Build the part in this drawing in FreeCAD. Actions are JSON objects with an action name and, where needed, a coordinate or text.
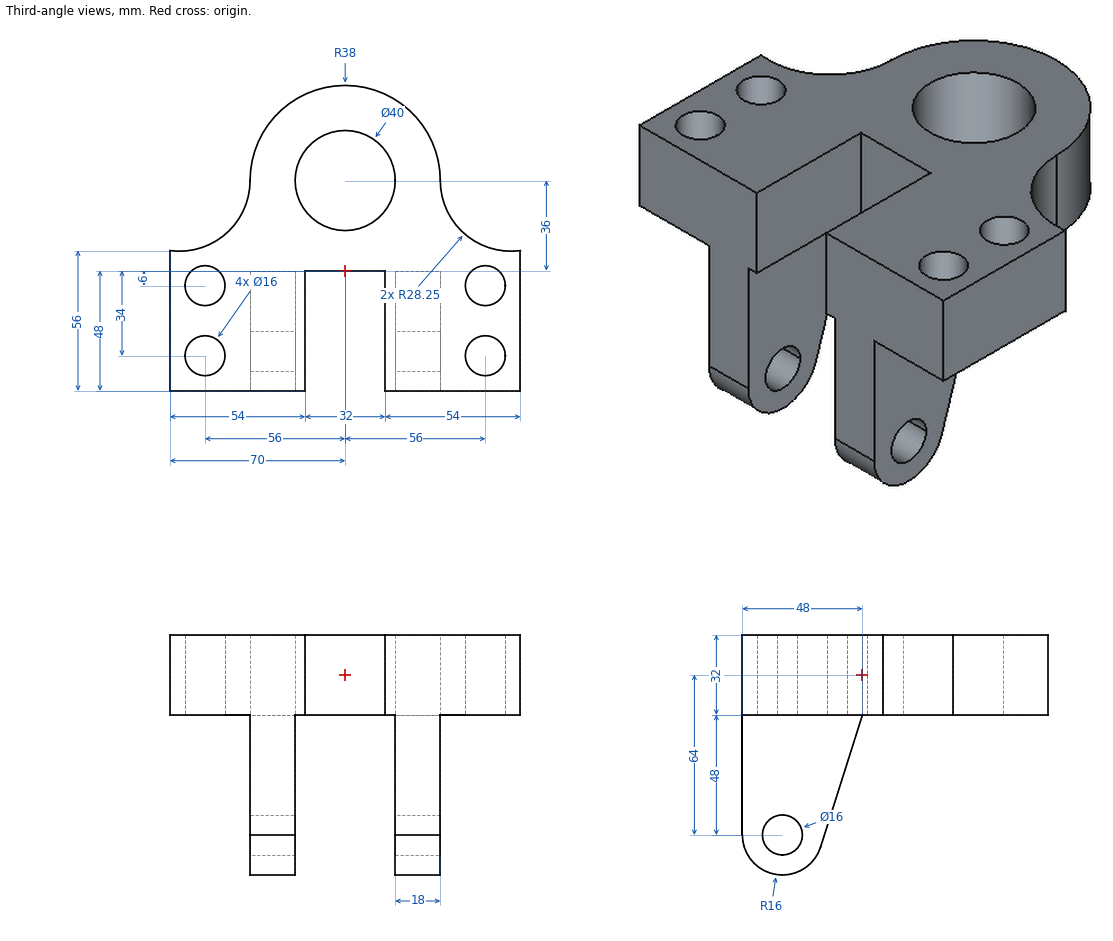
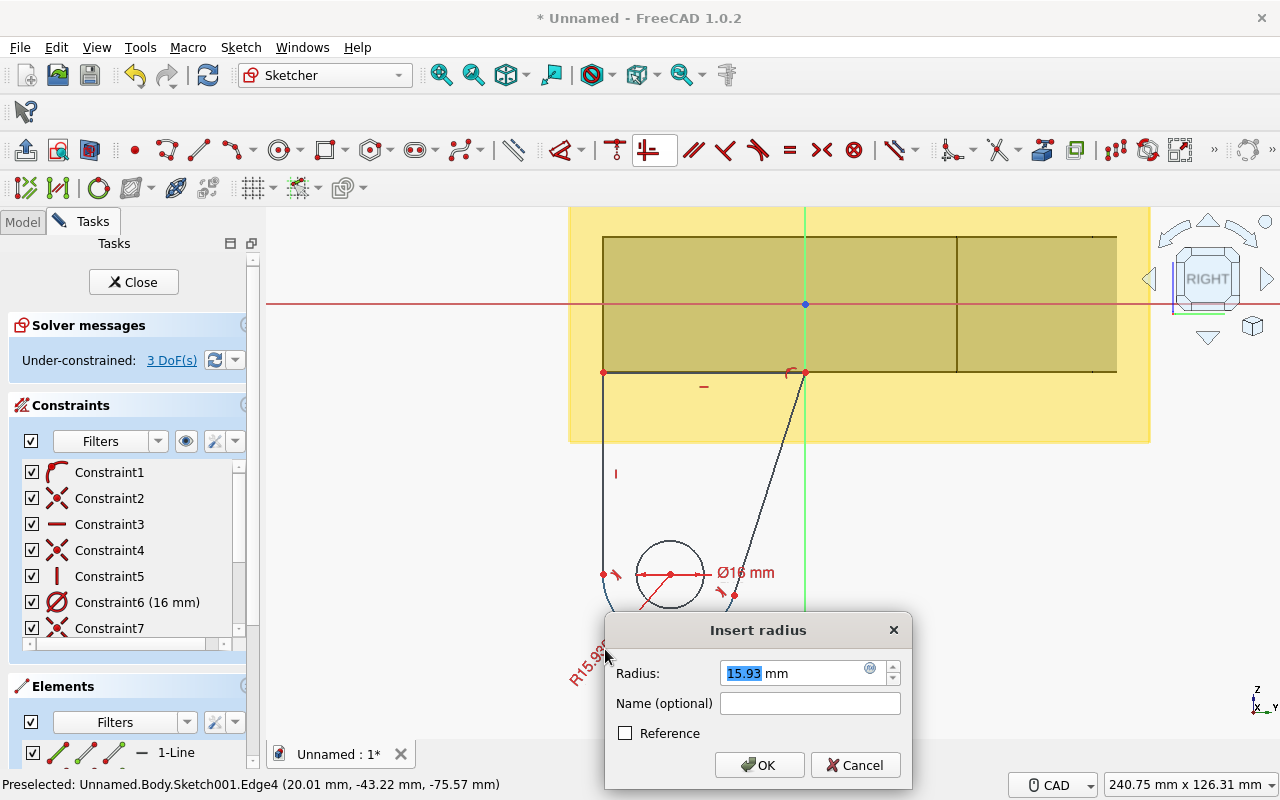
{"action": "type", "text": "16"}
{"action": "key", "text": "Return"}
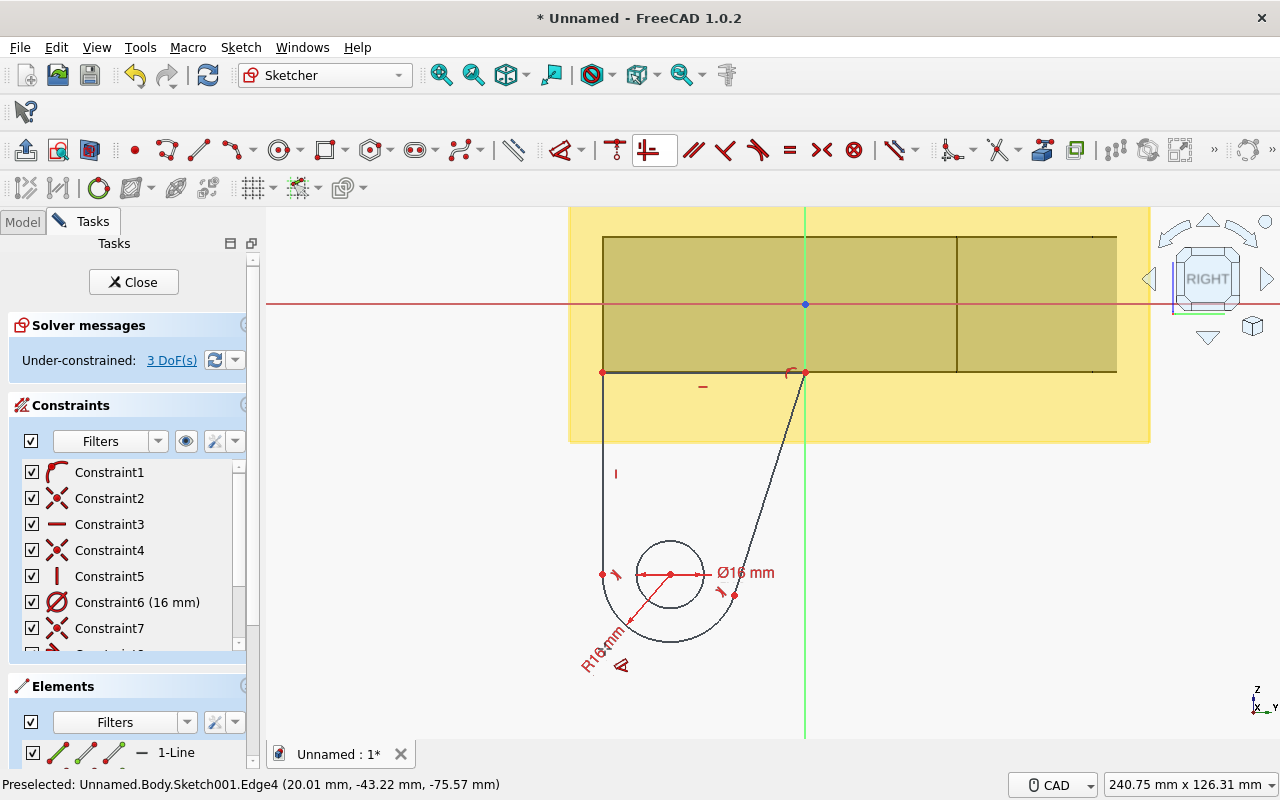
{"action": "left_click", "coordinate": [744, 373]}
{"action": "left_click", "coordinate": [704, 339]}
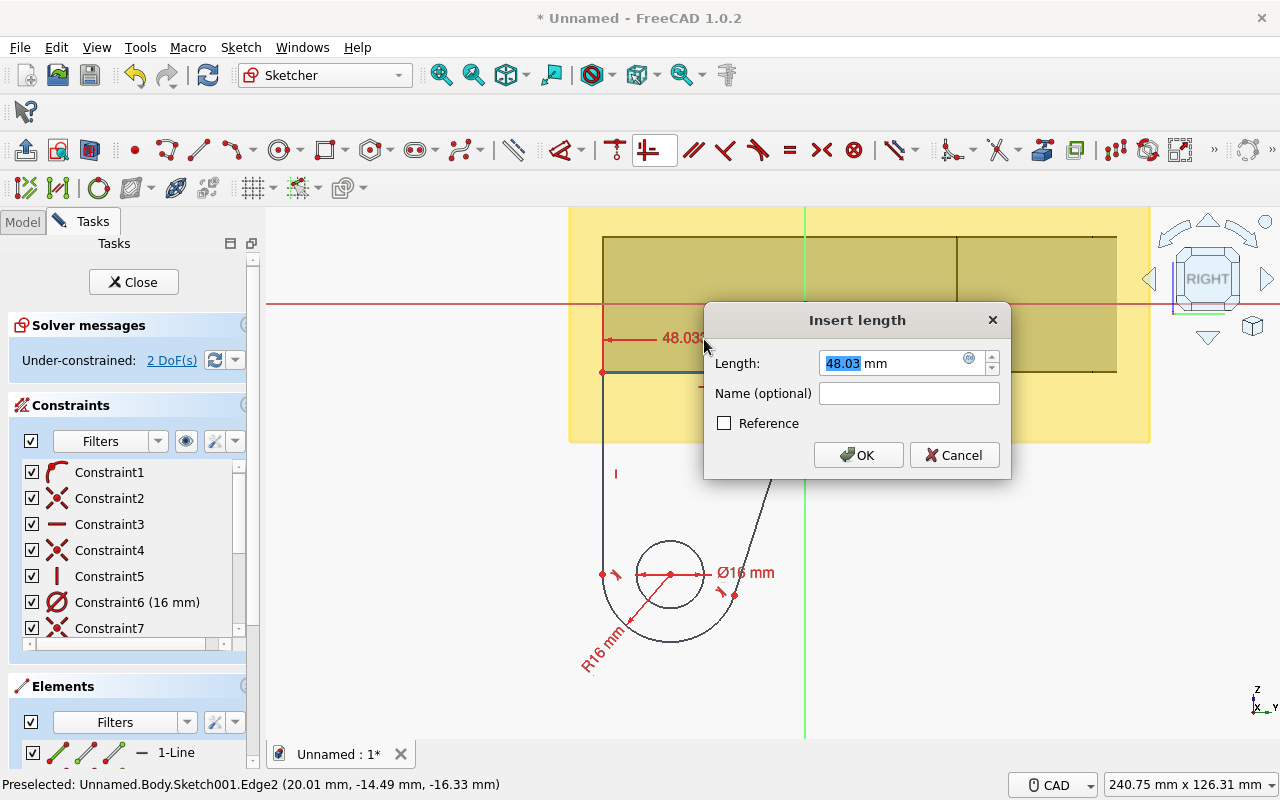
{"action": "type", "text": "48"}
{"action": "key", "text": "Return"}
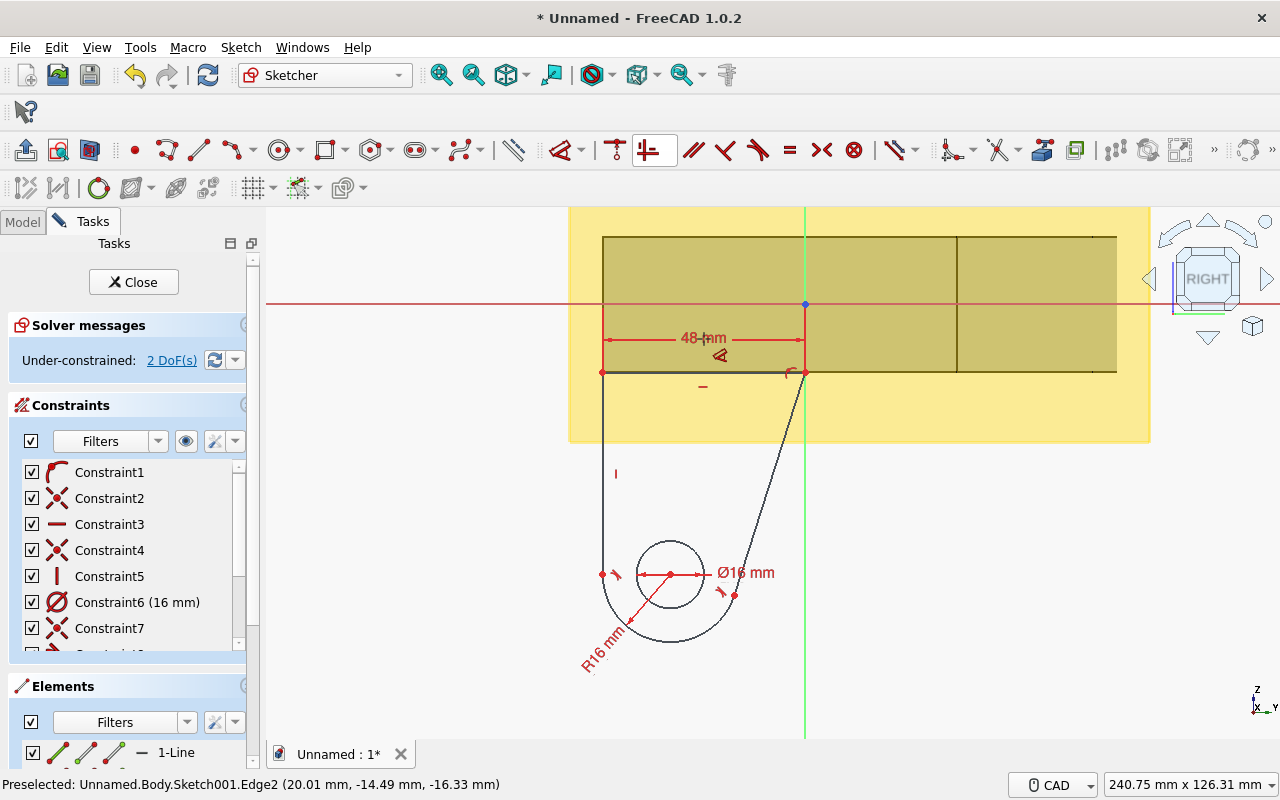
{"action": "left_click", "coordinate": [603, 434]}
{"action": "left_click", "coordinate": [569, 474]}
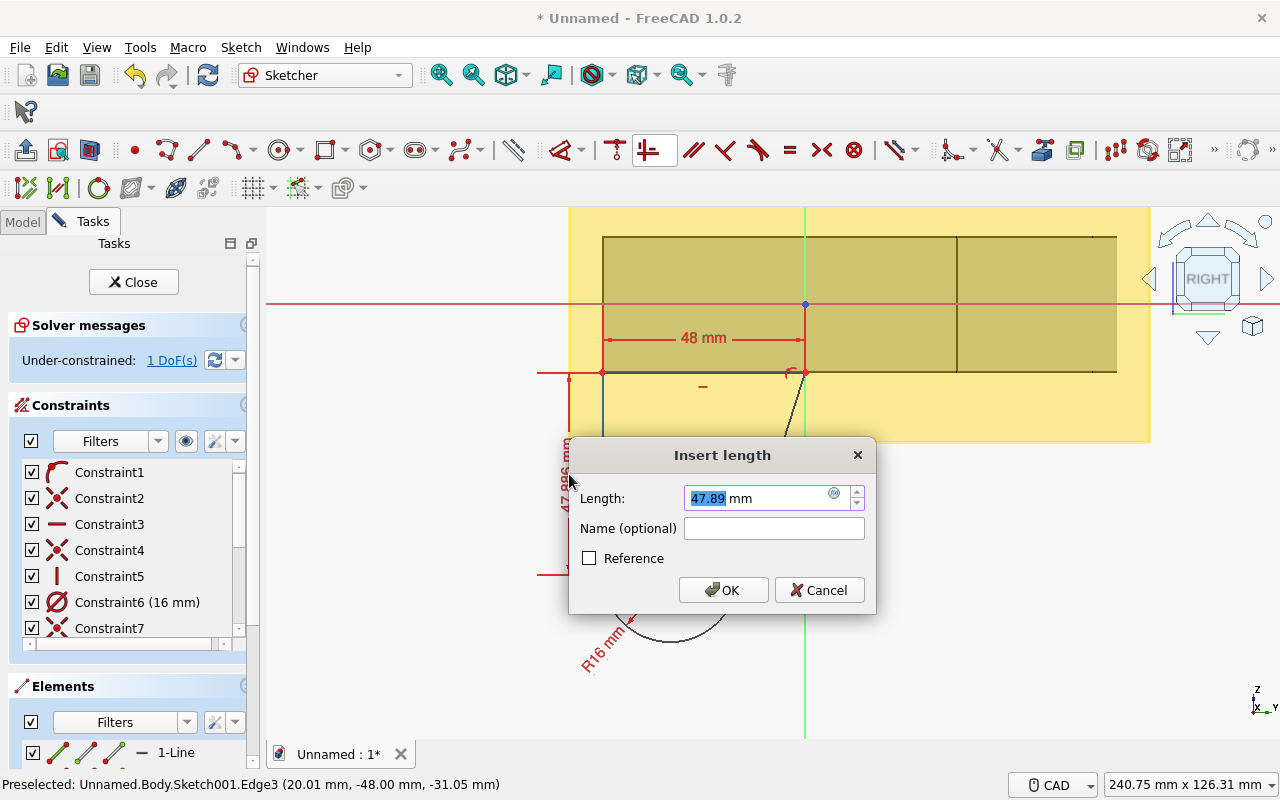
{"action": "type", "text": "48"}
{"action": "key", "text": "Return"}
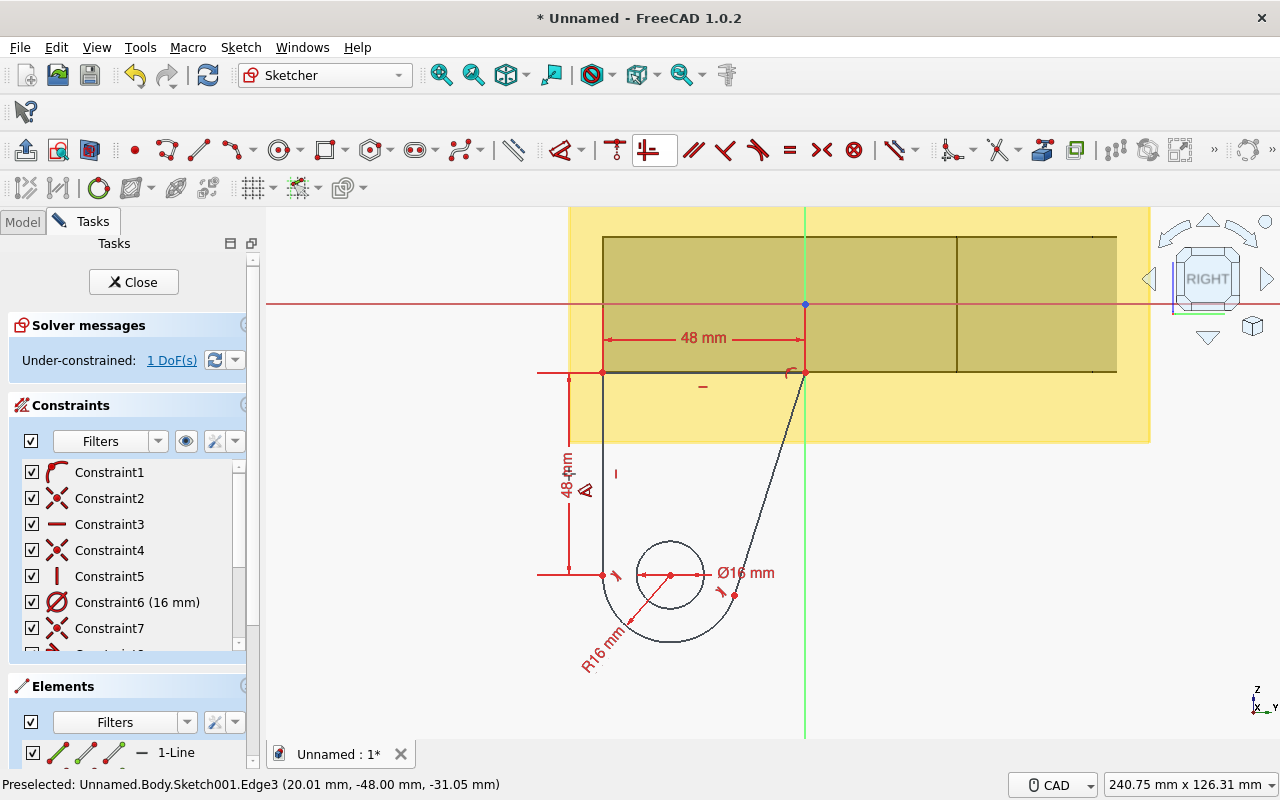
{"action": "left_click", "coordinate": [670, 575]}
{"action": "left_click", "coordinate": [839, 440]}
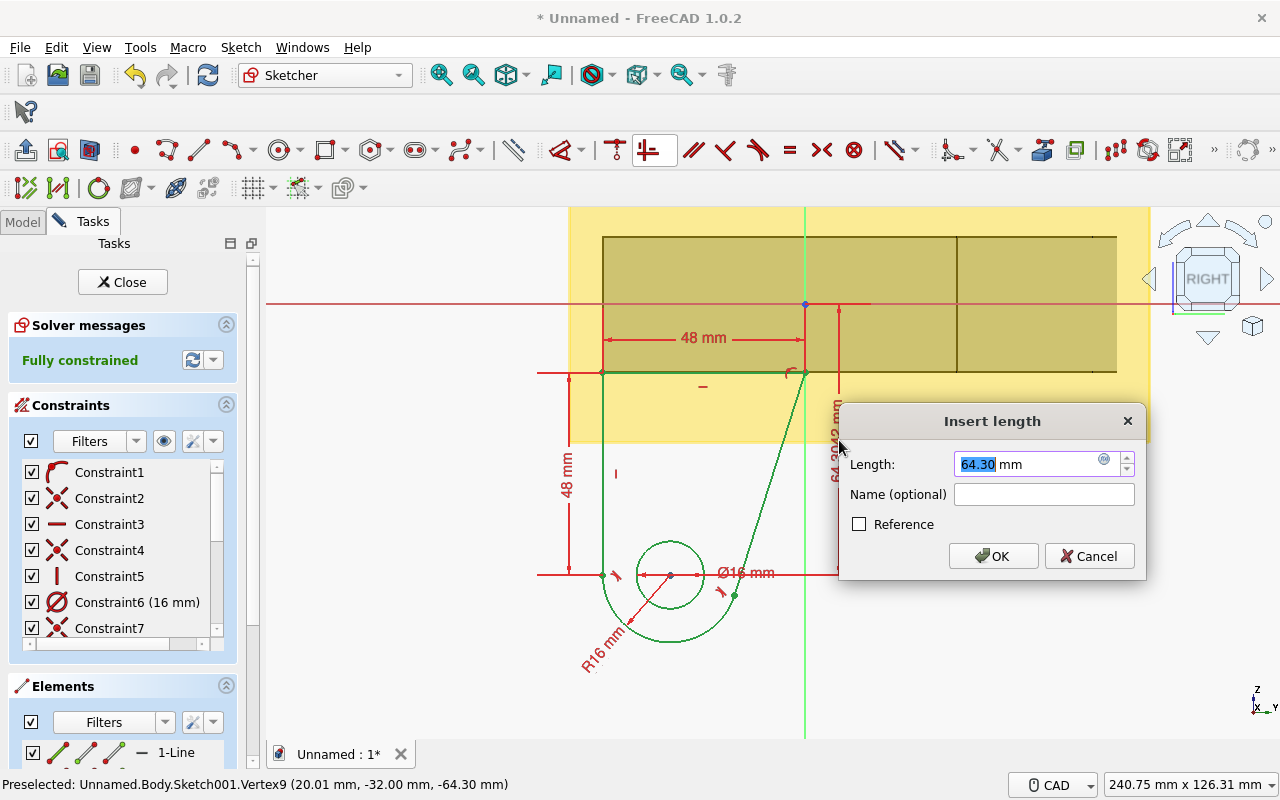
{"action": "type", "text": "64"}
{"action": "key", "text": "Return"}
{"action": "key", "text": "Escape"}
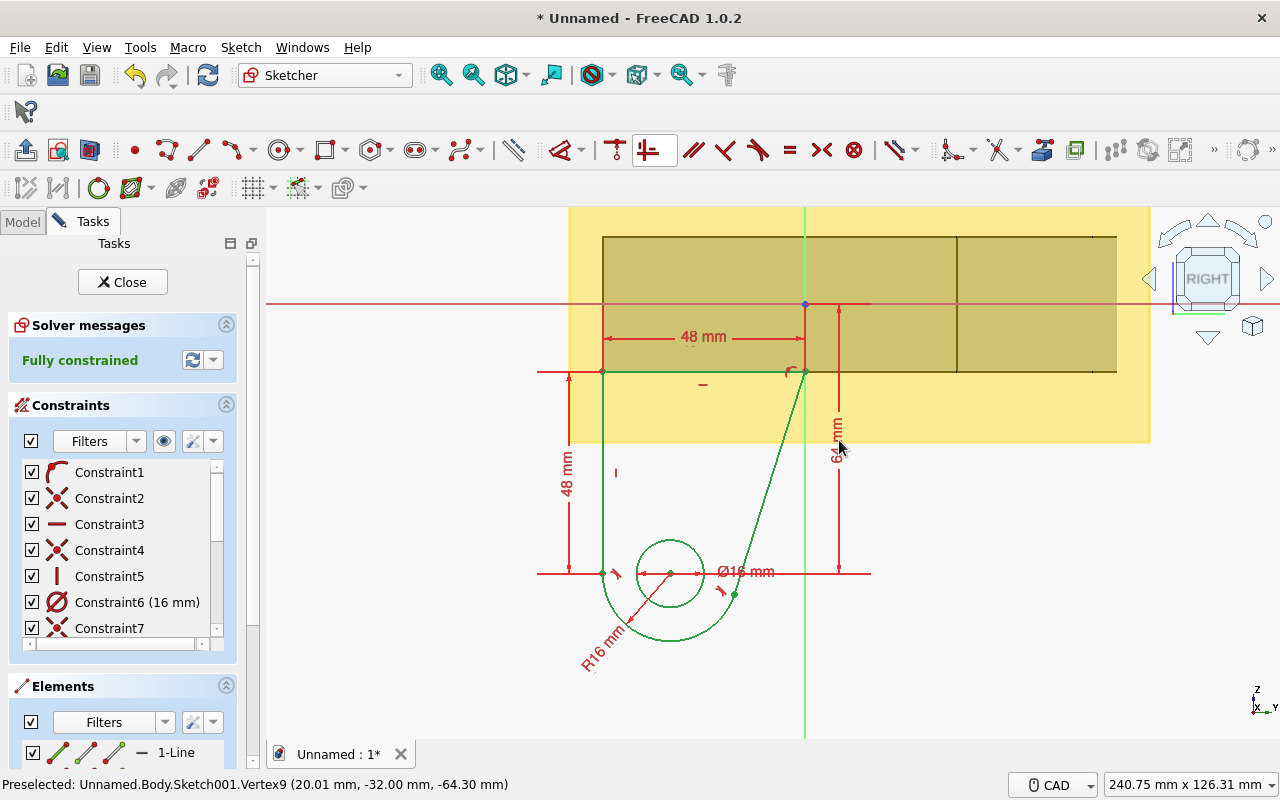
{"action": "left_click", "coordinate": [123, 282]}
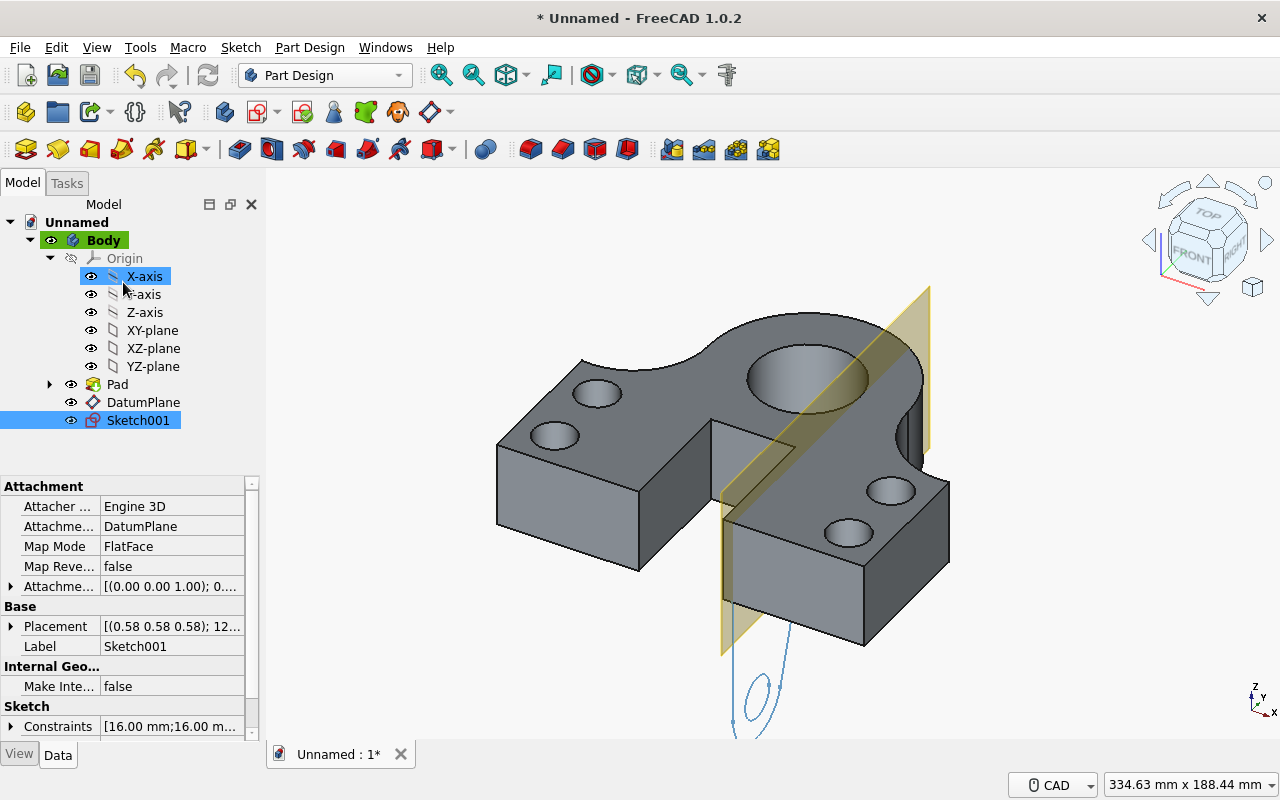
{"action": "left_click", "coordinate": [26, 150]}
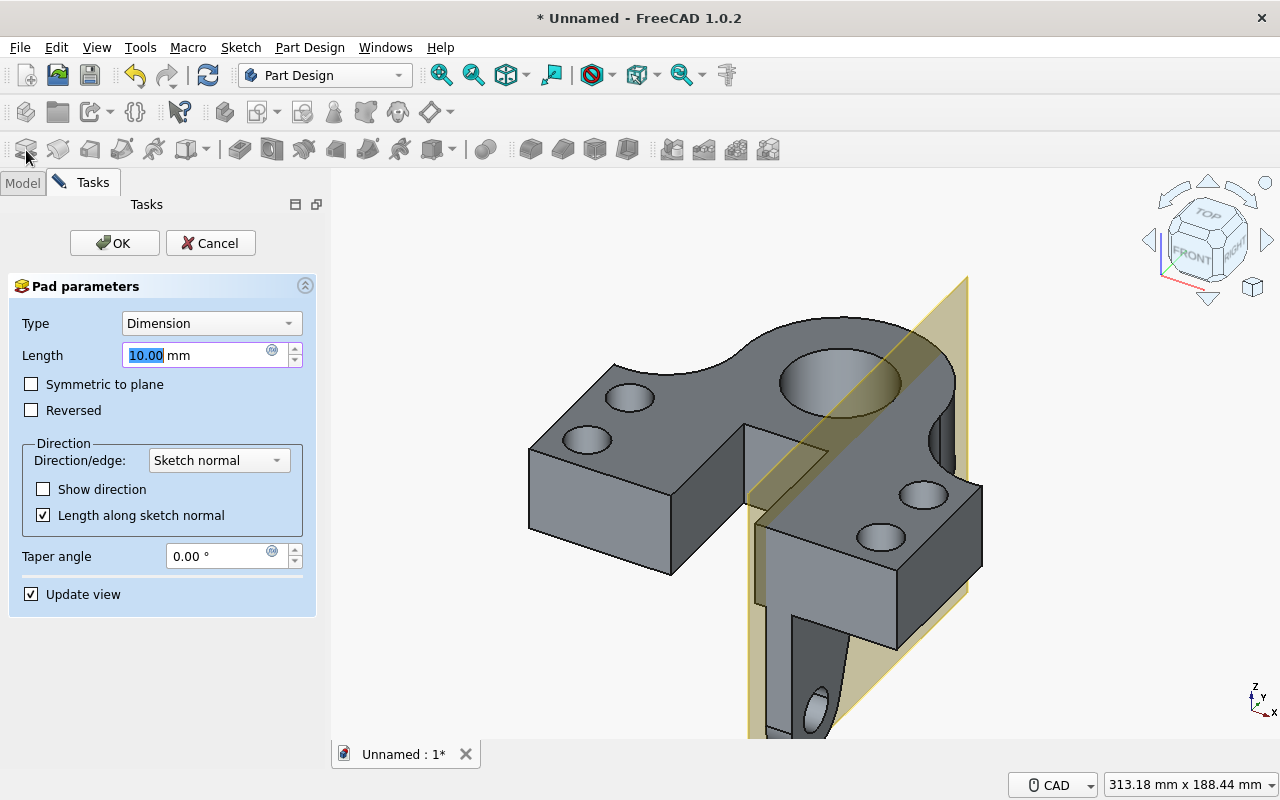
{"action": "type", "text": "18"}
{"action": "key", "text": "Tab"}